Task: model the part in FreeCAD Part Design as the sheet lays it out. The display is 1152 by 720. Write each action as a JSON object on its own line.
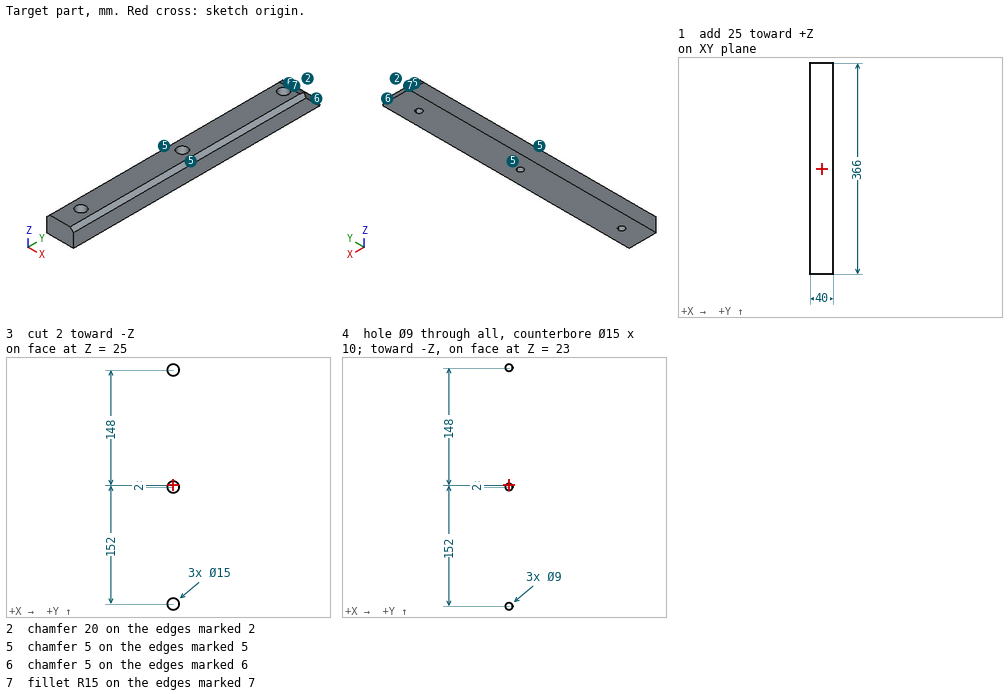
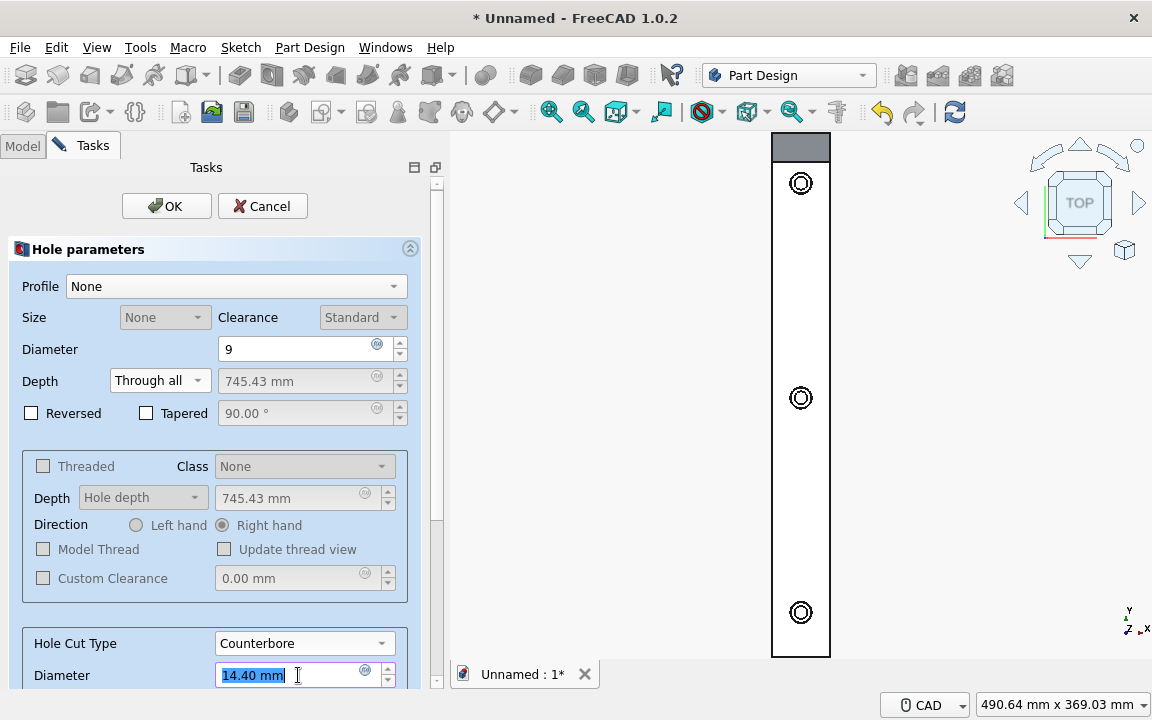
{"action": "type", "text": "15"}
{"action": "key", "text": "Tab"}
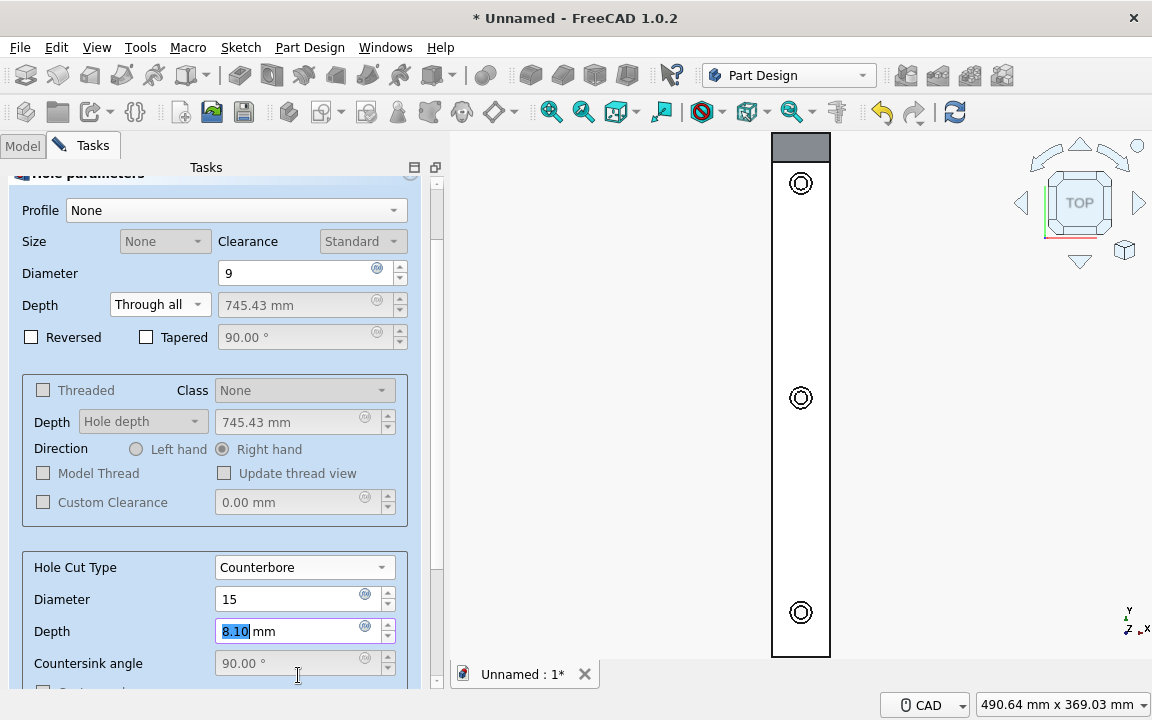
{"action": "type", "text": "10"}
{"action": "key", "text": "Tab"}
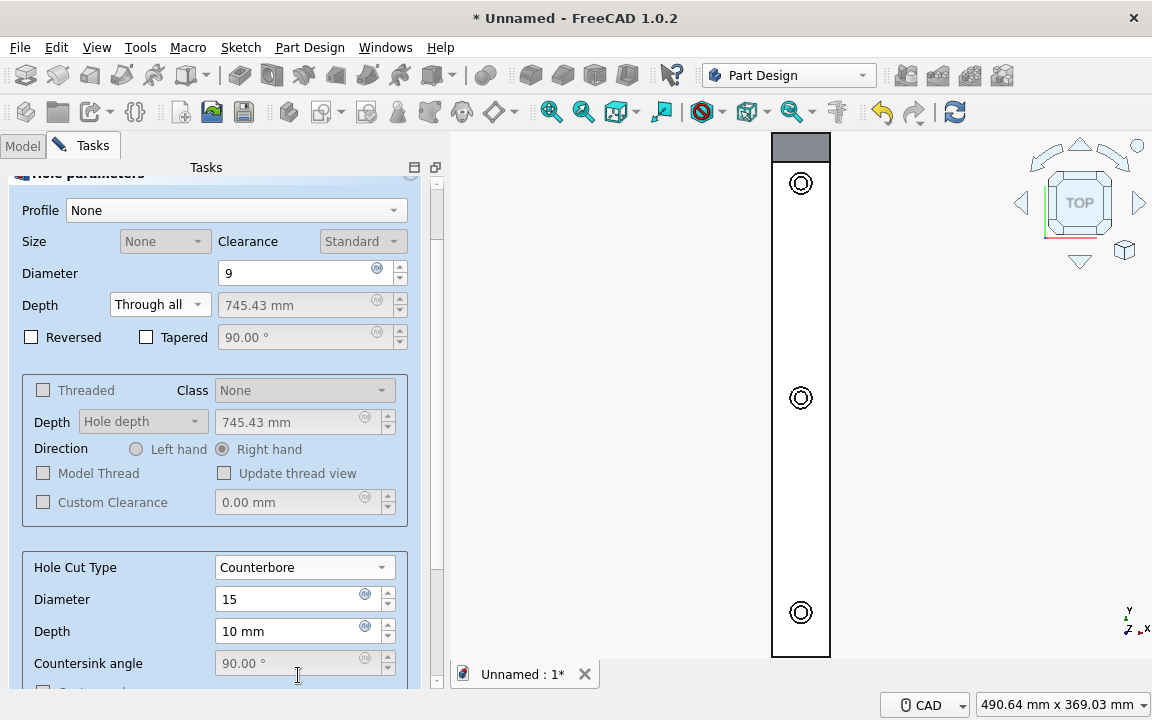
{"action": "scroll", "coordinate": [437, 432], "scroll_direction": "up", "scroll_amount": 3}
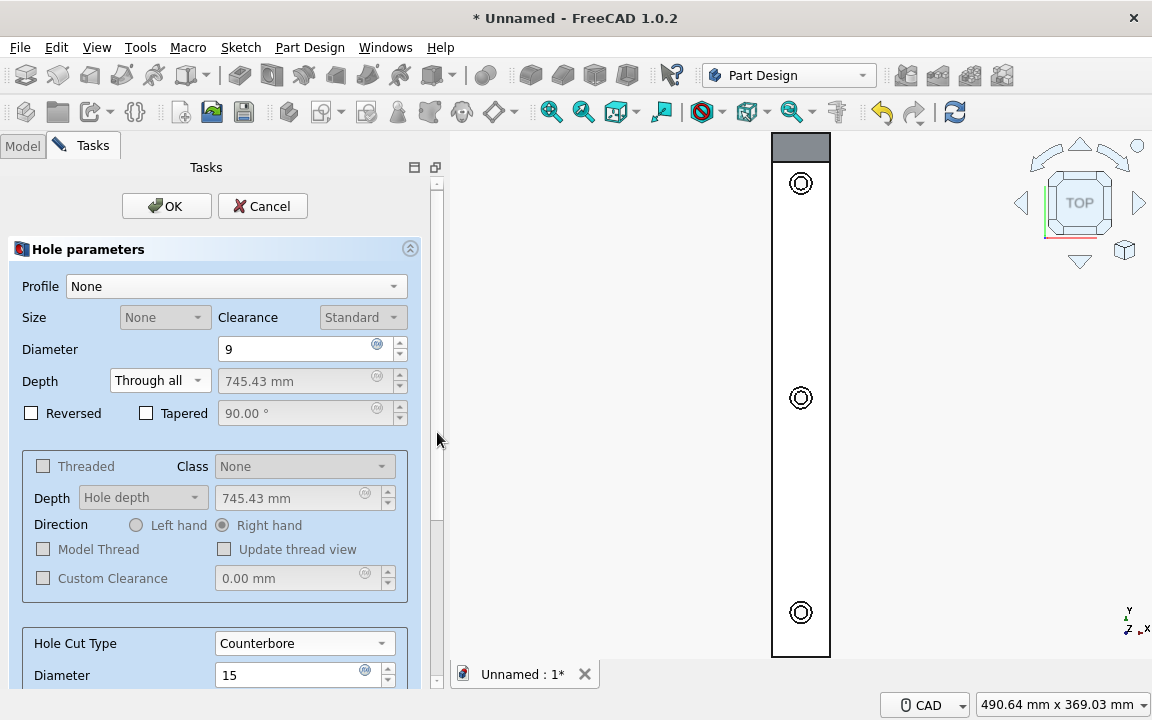
{"action": "left_click", "coordinate": [167, 206]}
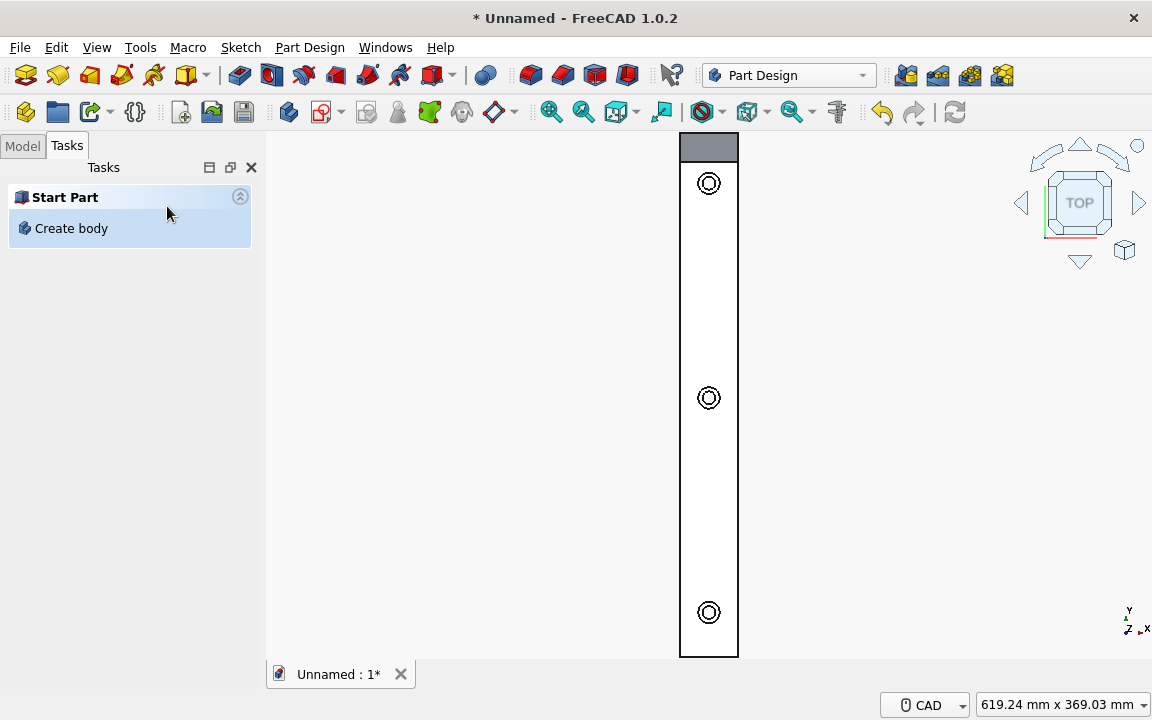
{"action": "left_click", "coordinate": [680, 408]}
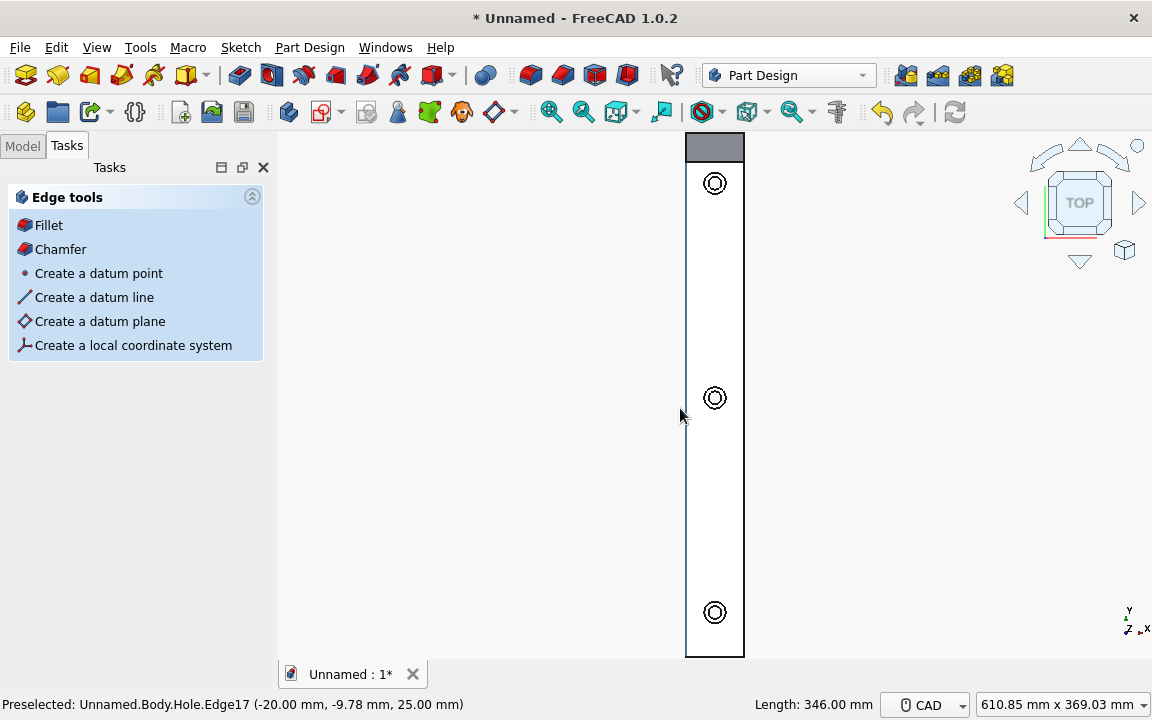
{"action": "left_click", "coordinate": [744, 408], "text": "ctrl"}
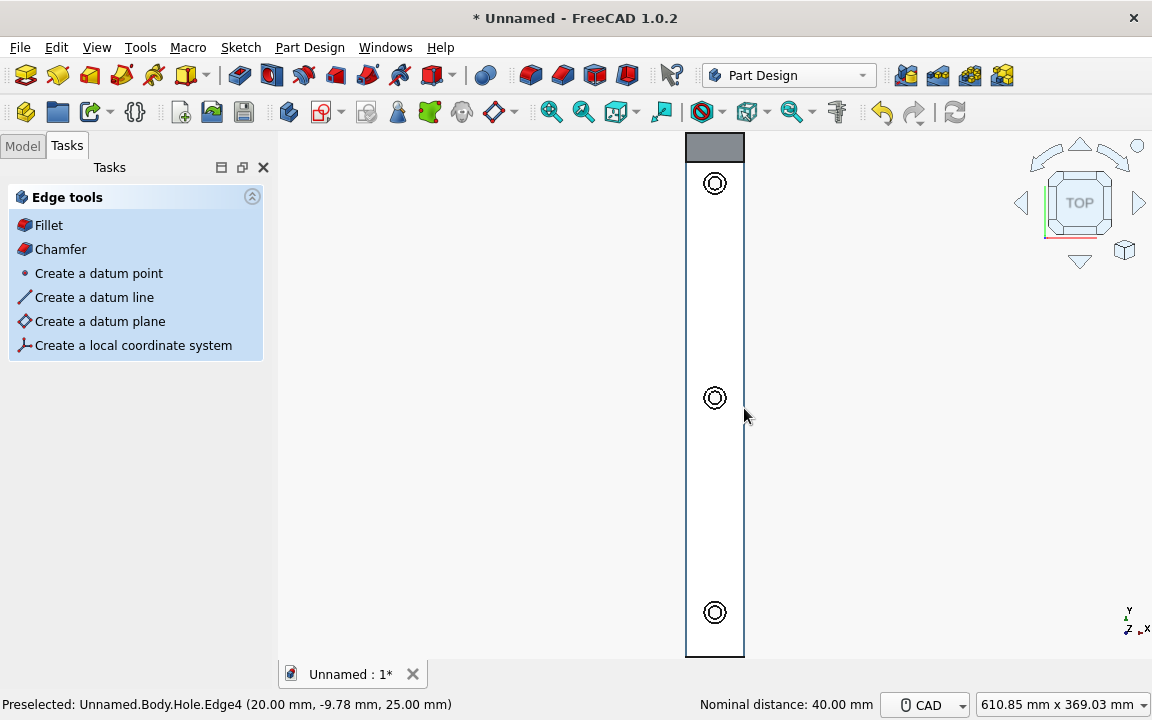
{"action": "left_click", "coordinate": [564, 76]}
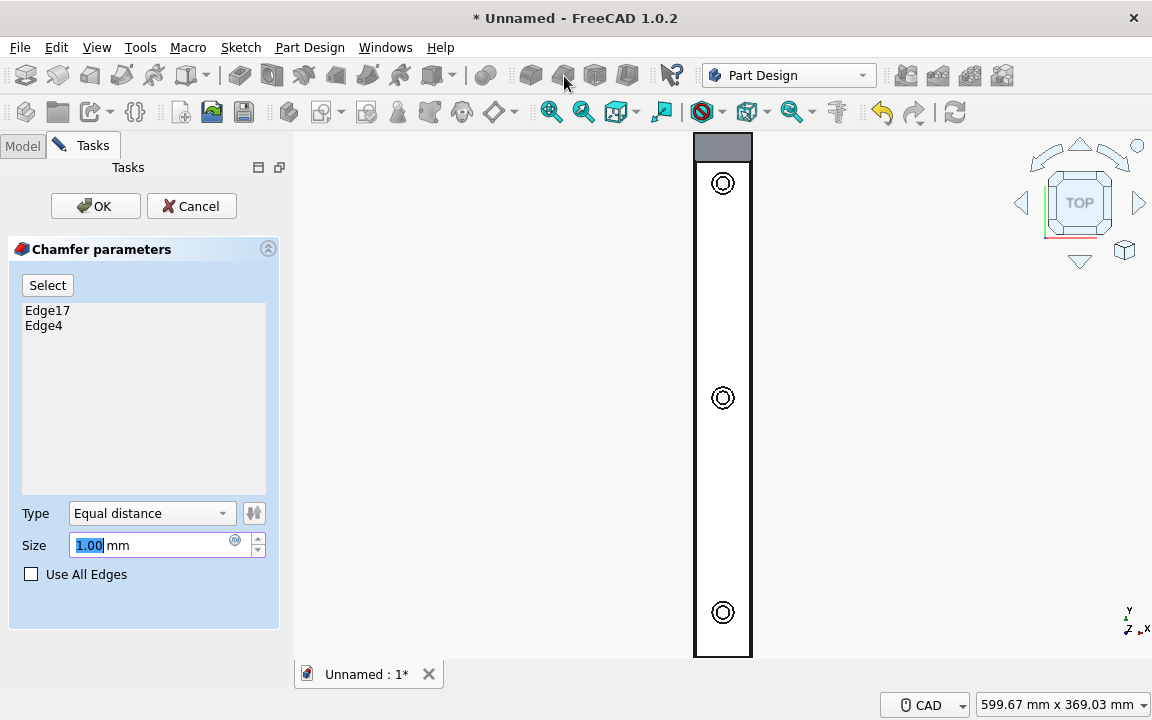
{"action": "type", "text": "5"}
{"action": "key", "text": "Tab"}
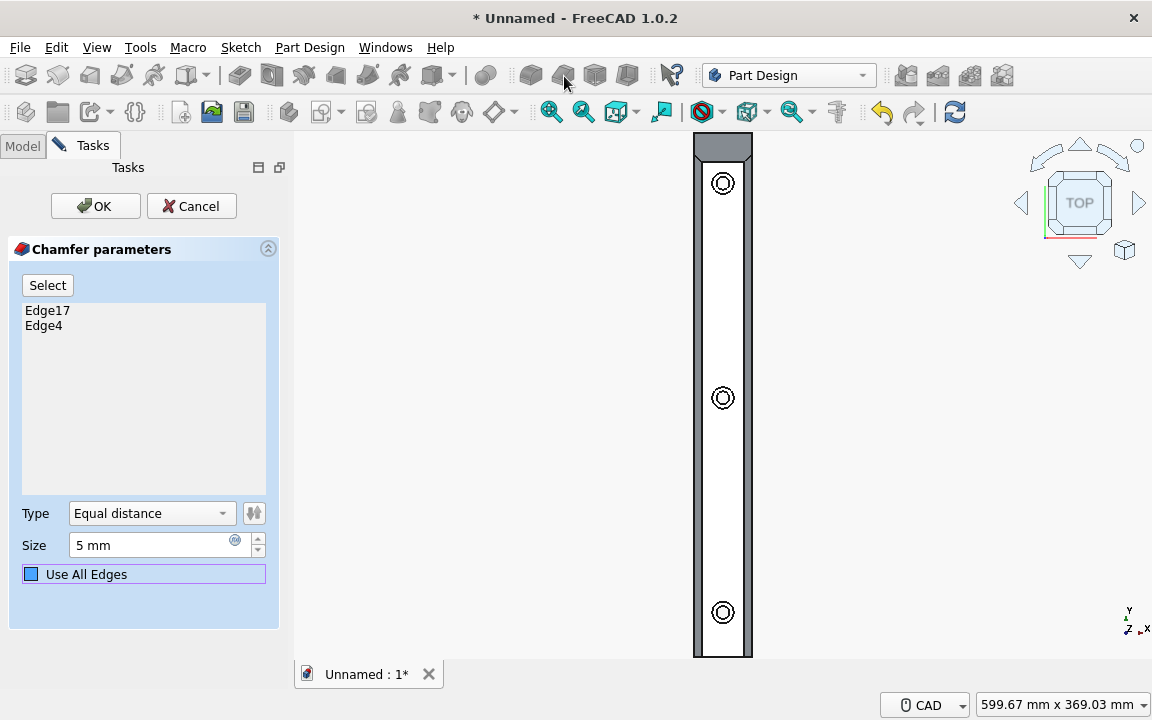
{"action": "left_click", "coordinate": [96, 206]}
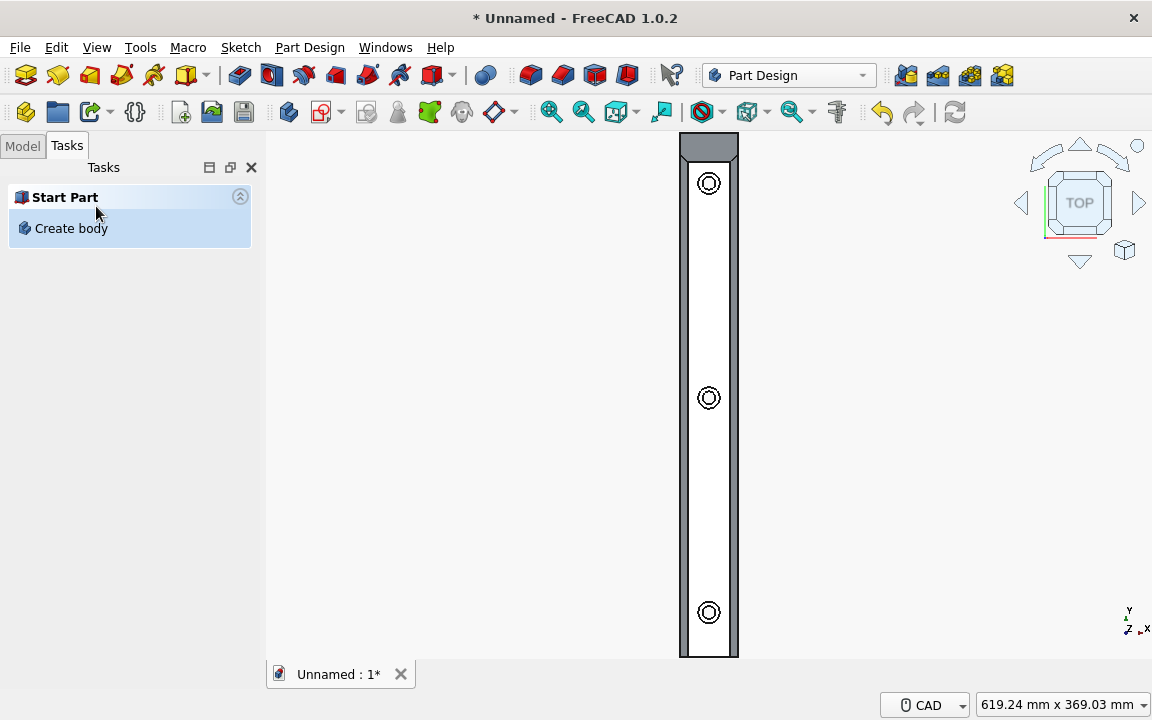
{"action": "key", "text": "0"}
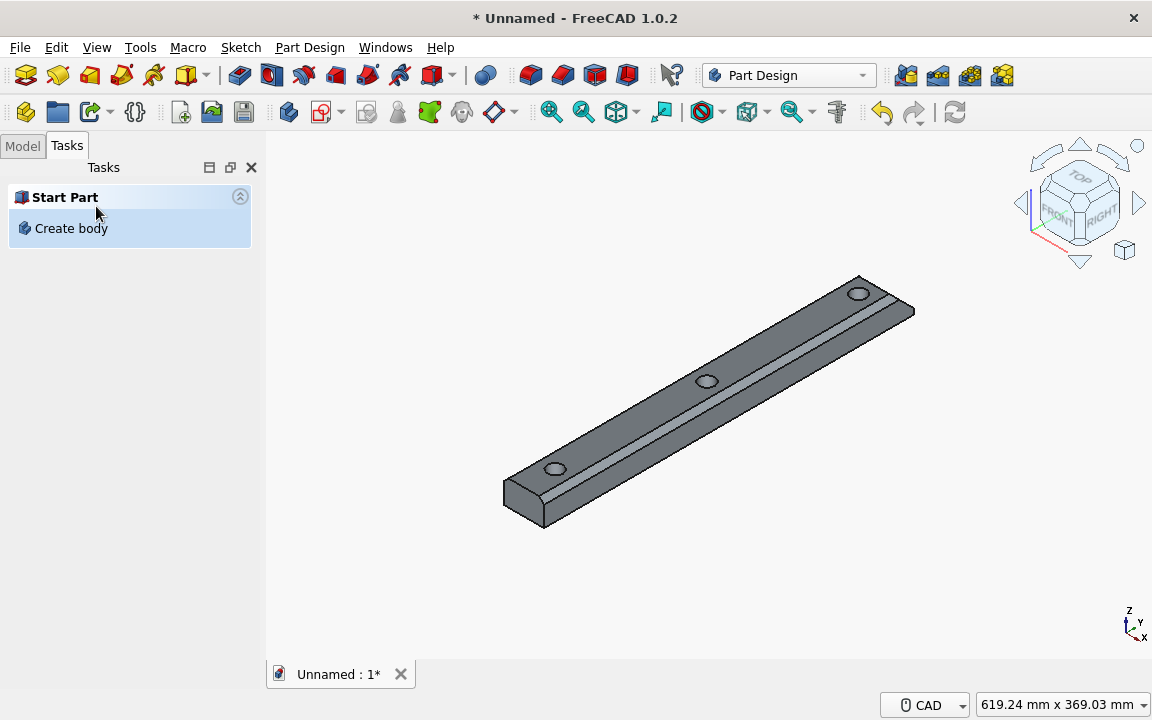
{"action": "key", "text": "2"}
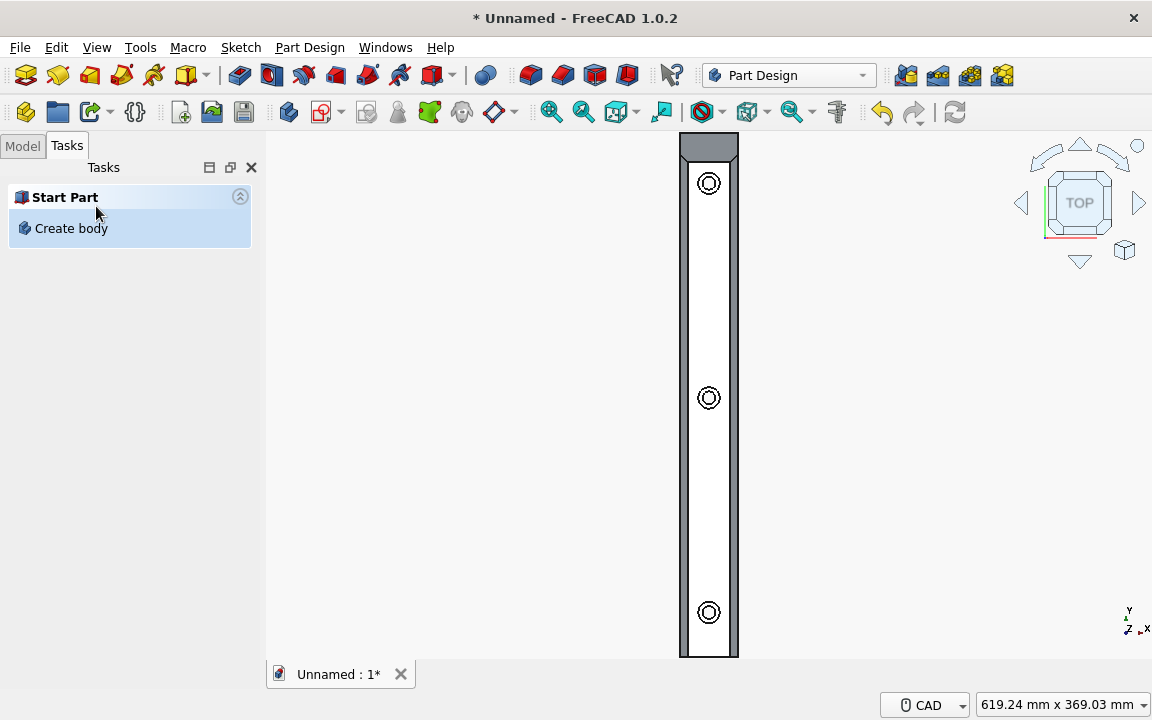
{"action": "key", "text": "1"}